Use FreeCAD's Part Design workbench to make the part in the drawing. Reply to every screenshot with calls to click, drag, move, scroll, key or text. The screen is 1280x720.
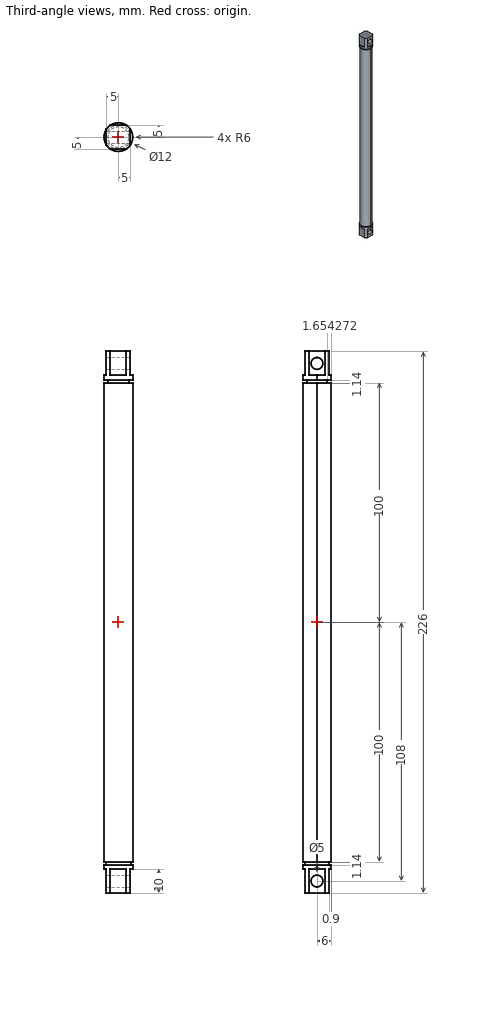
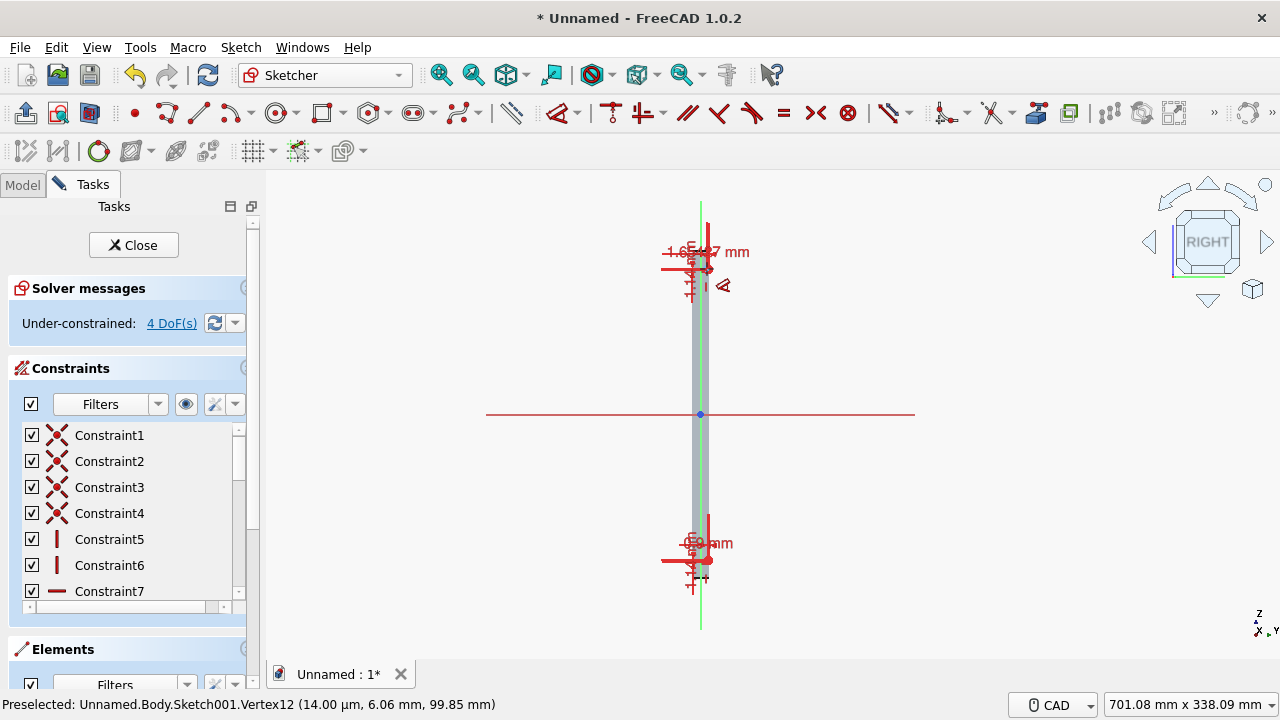
scroll(709, 562, up, 12)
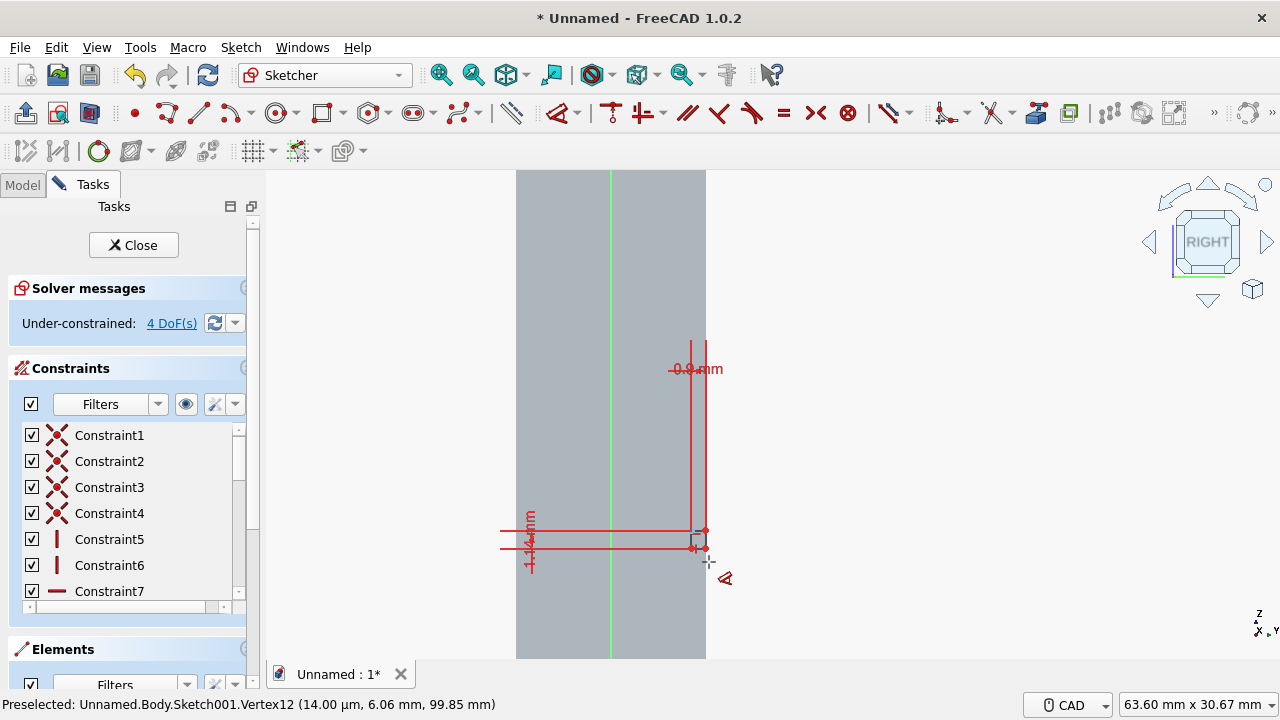
click(706, 549)
click(658, 583)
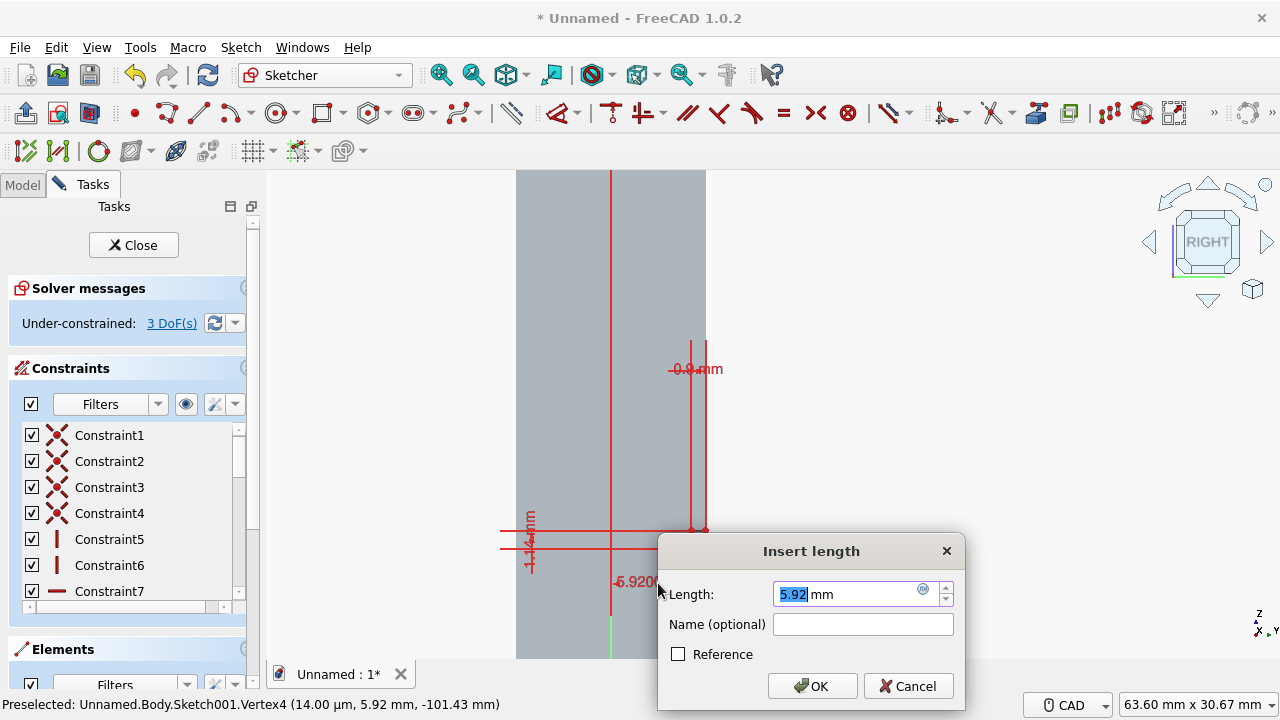
text(6)
key(Return)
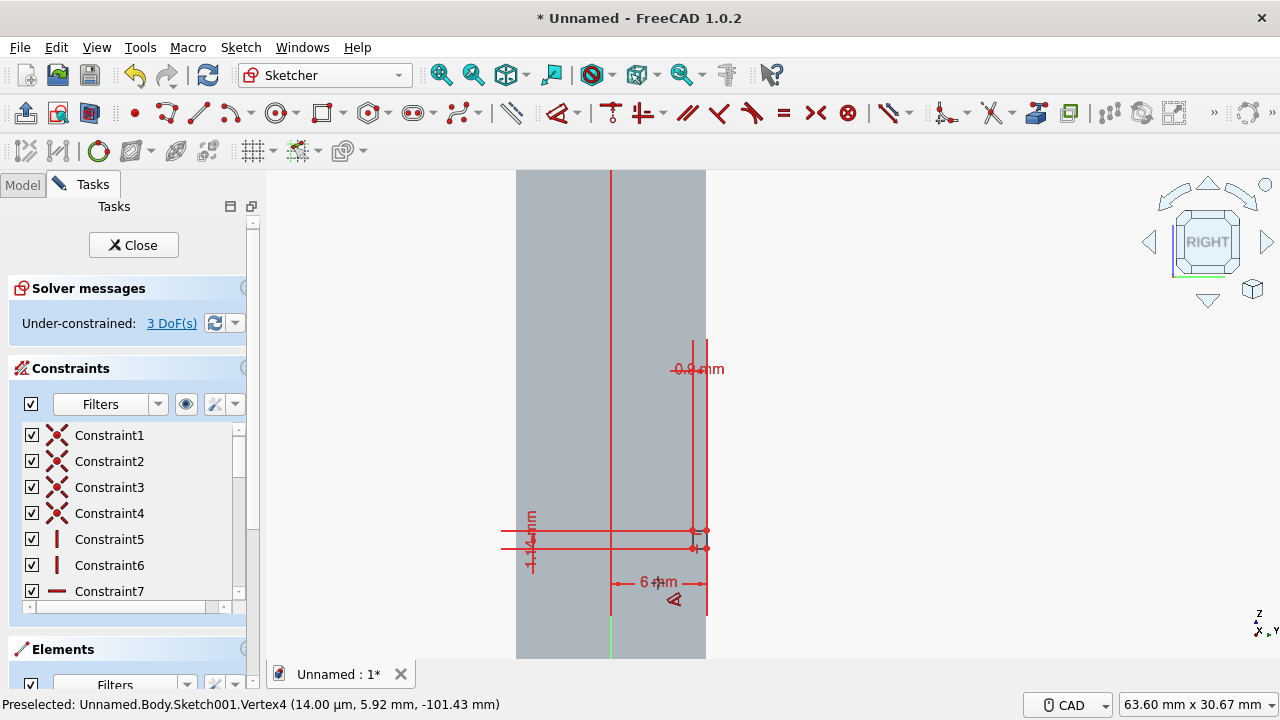
scroll(709, 562, down, 12)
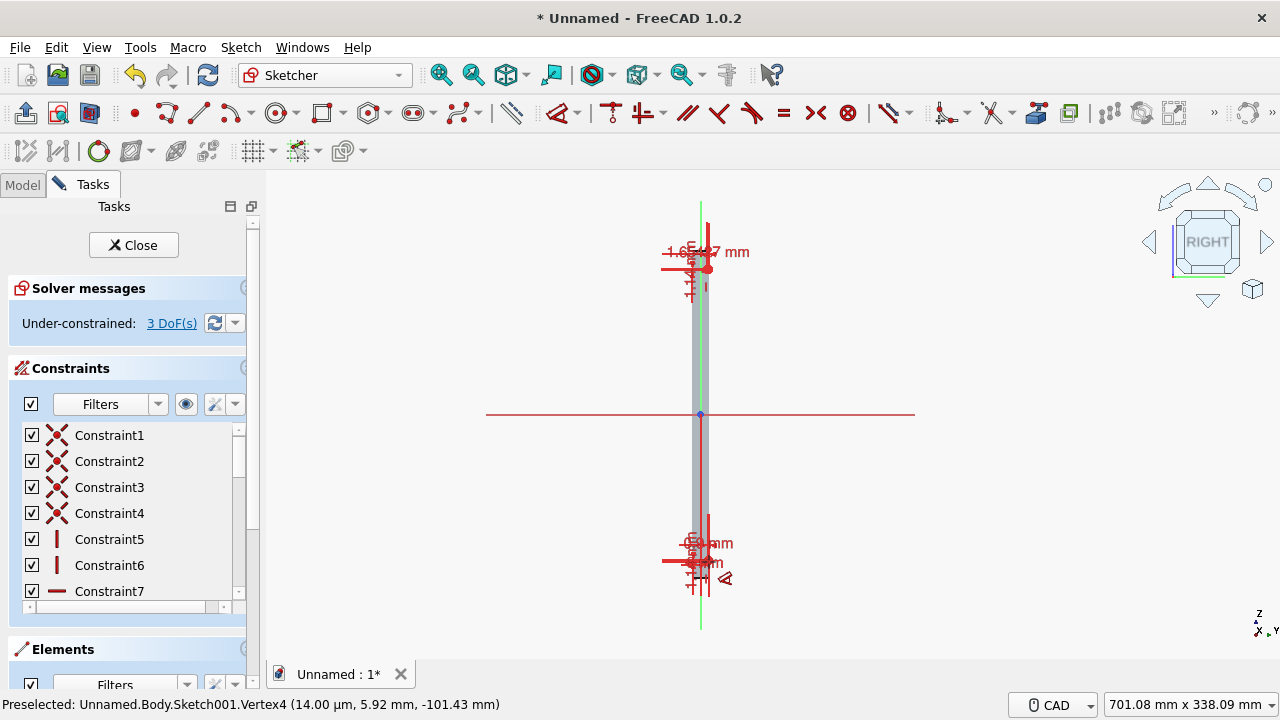
scroll(709, 270, up, 11)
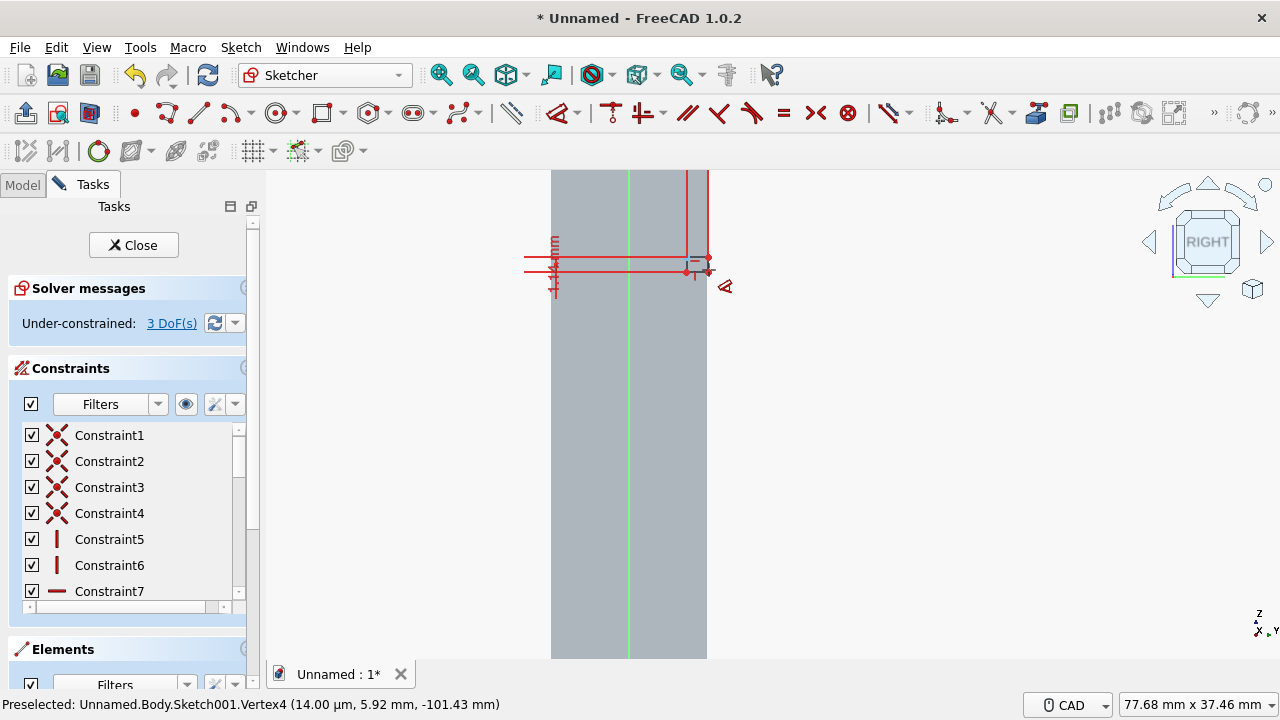
click(708, 272)
click(669, 238)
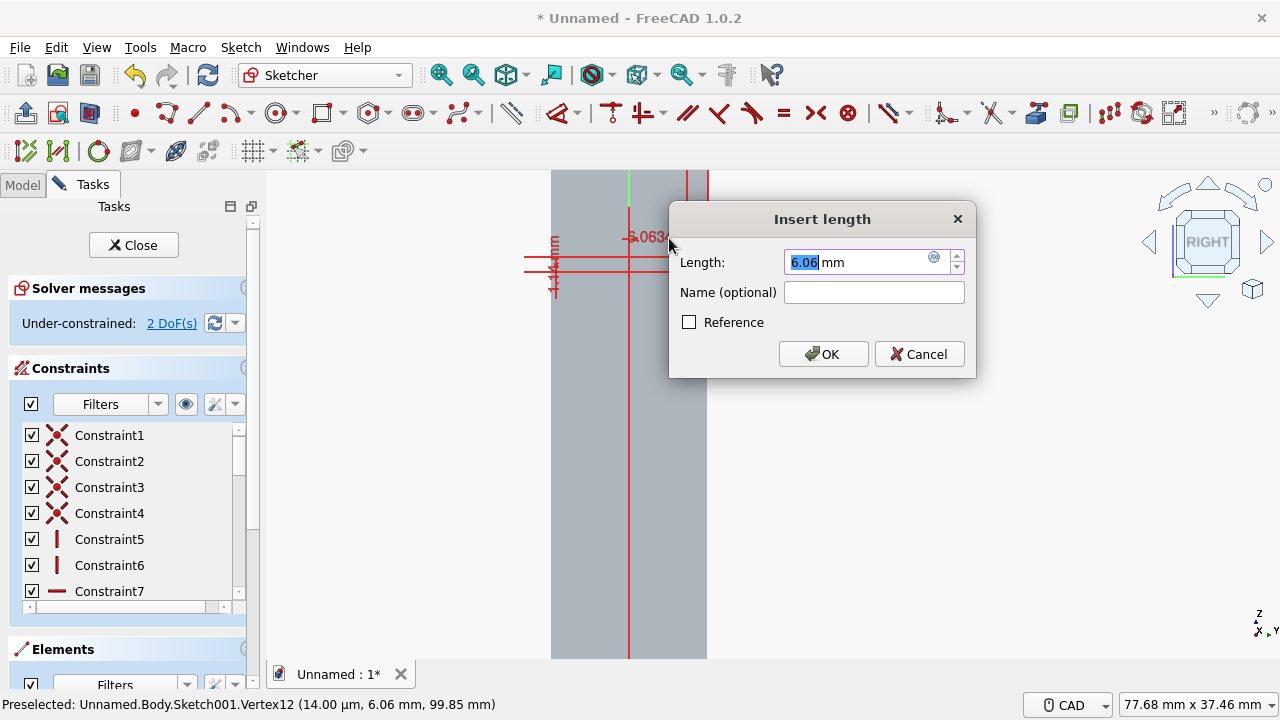
text(6)
key(Return)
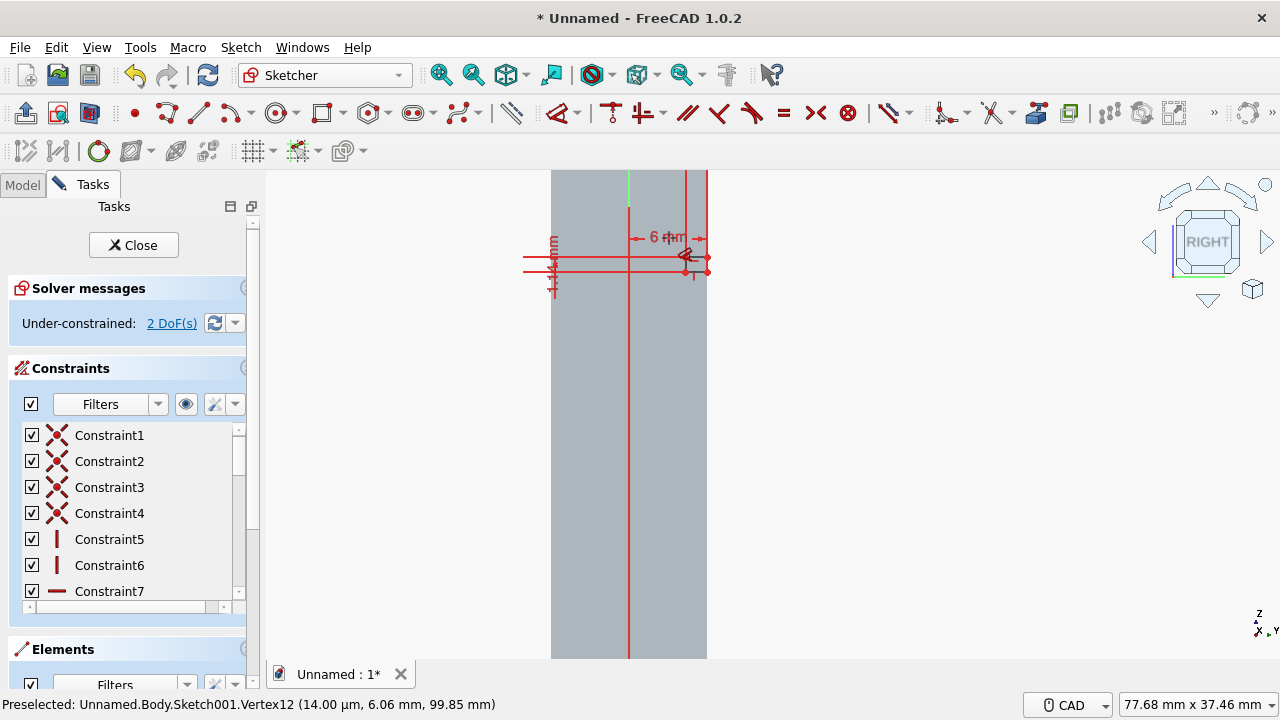
scroll(709, 270, down, 11)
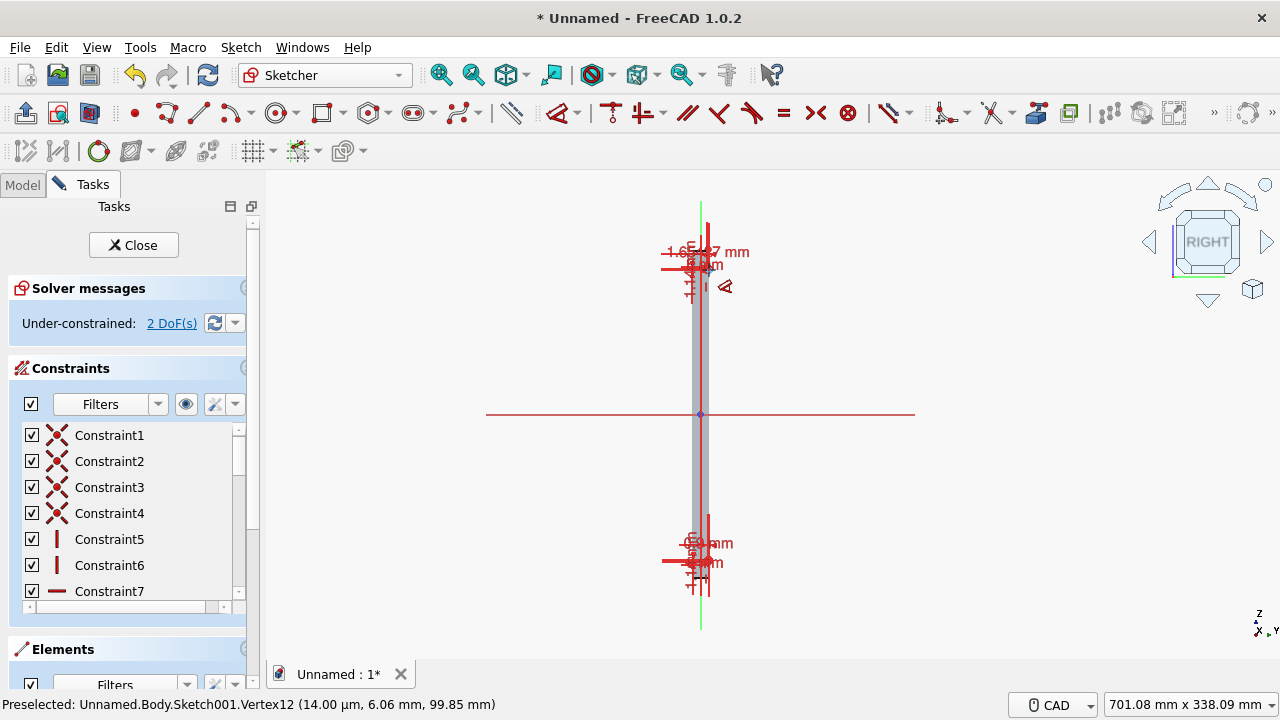
scroll(708, 560, up, 12)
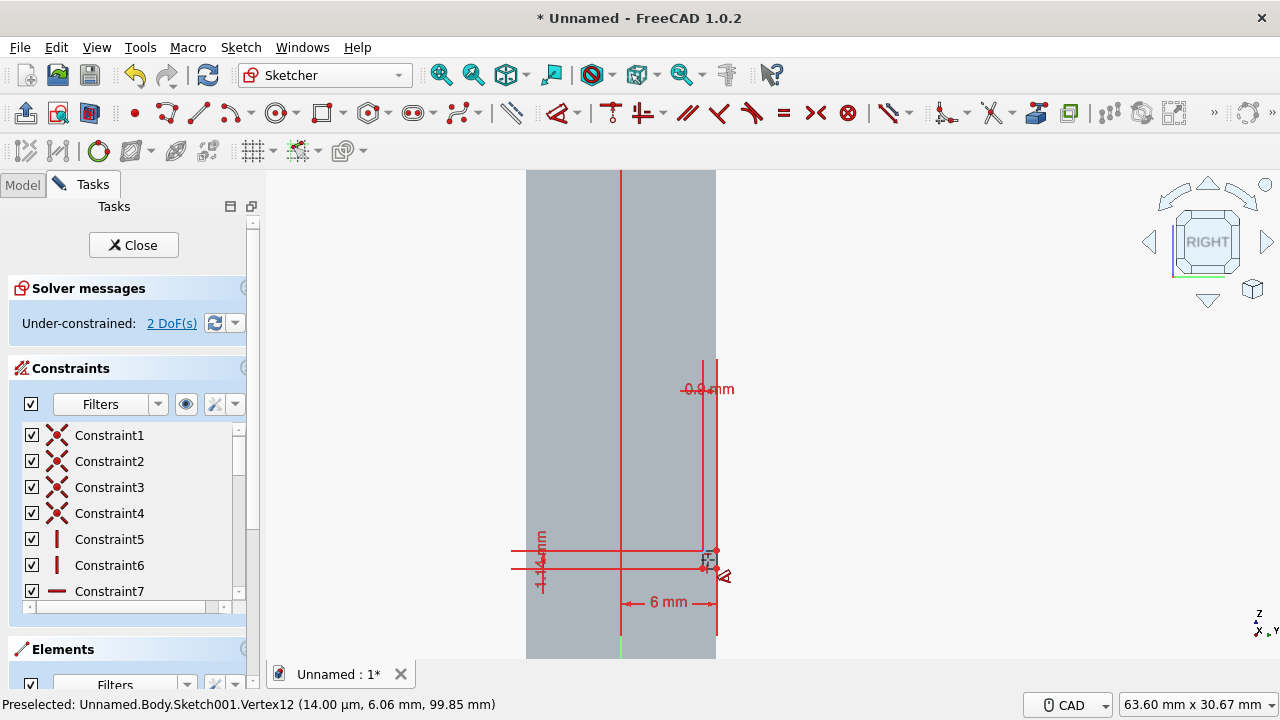
click(703, 551)
click(587, 374)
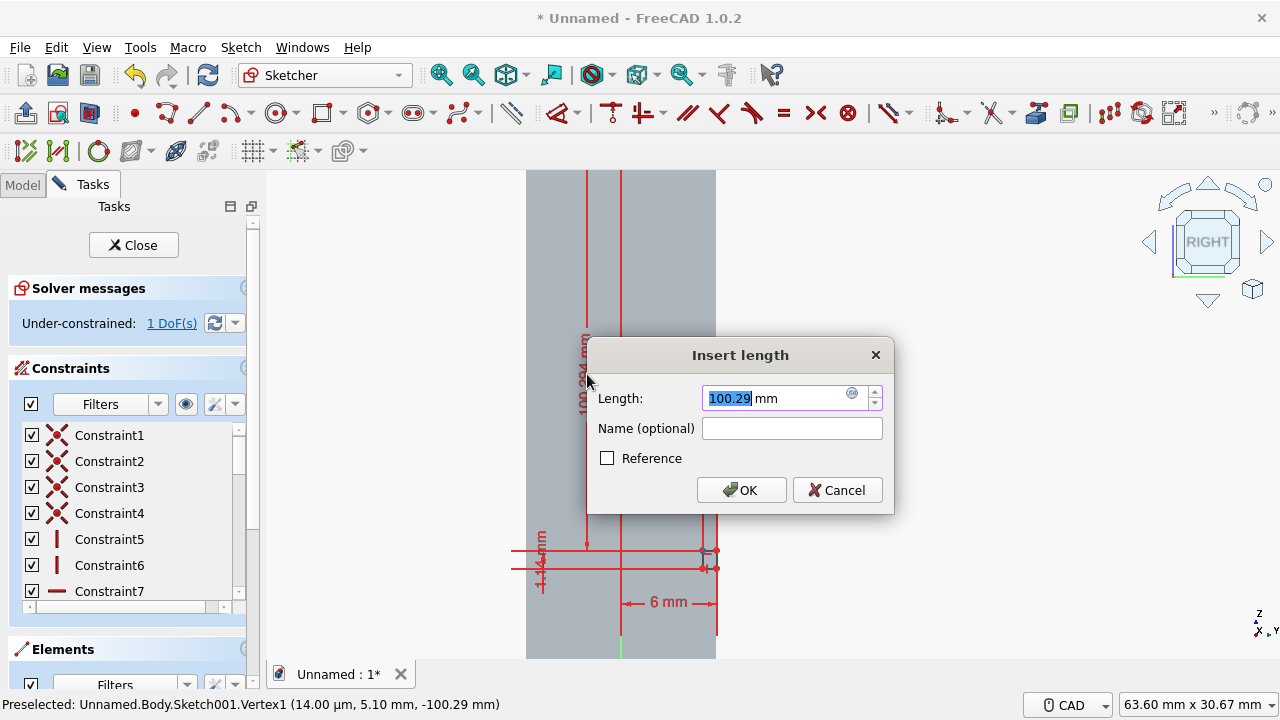
text(100)
key(Return)